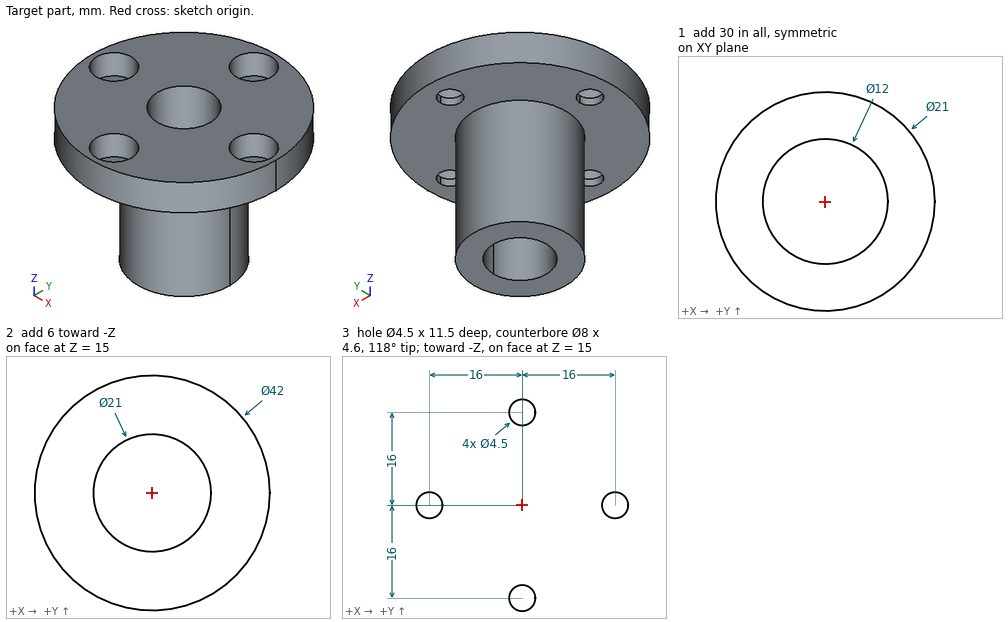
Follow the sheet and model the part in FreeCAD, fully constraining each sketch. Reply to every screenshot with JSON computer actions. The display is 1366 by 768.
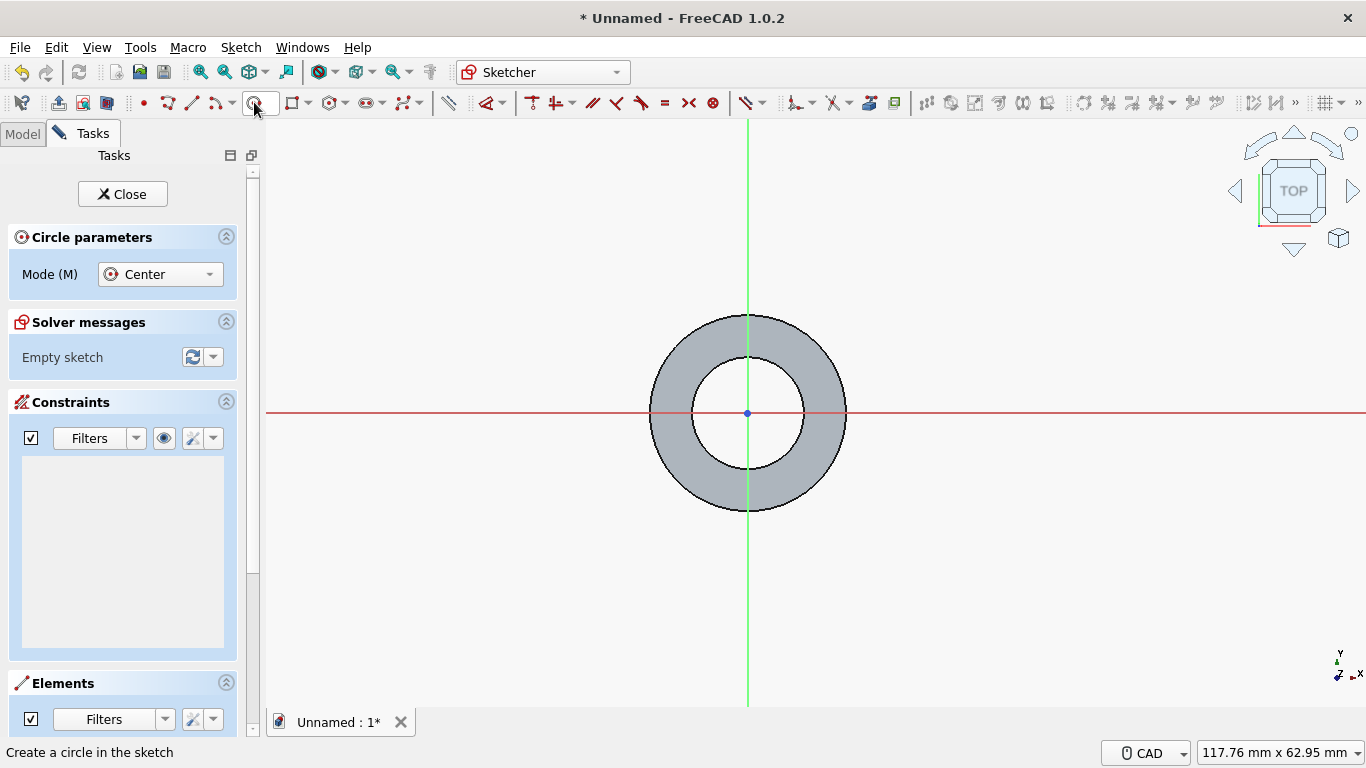
{"action": "left_click", "coordinate": [748, 413]}
{"action": "mouse_move", "coordinate": [887, 274]}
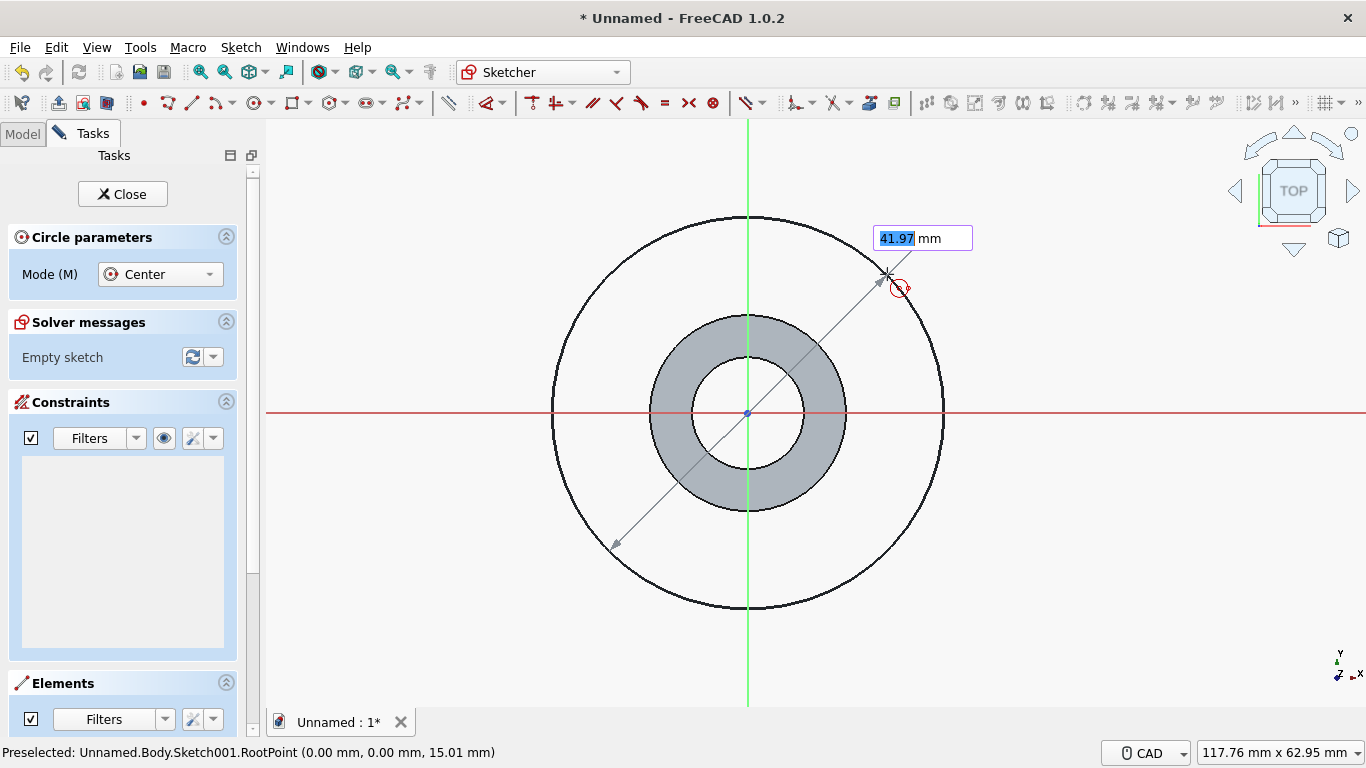
{"action": "type", "text": "42"}
{"action": "key", "text": "Return"}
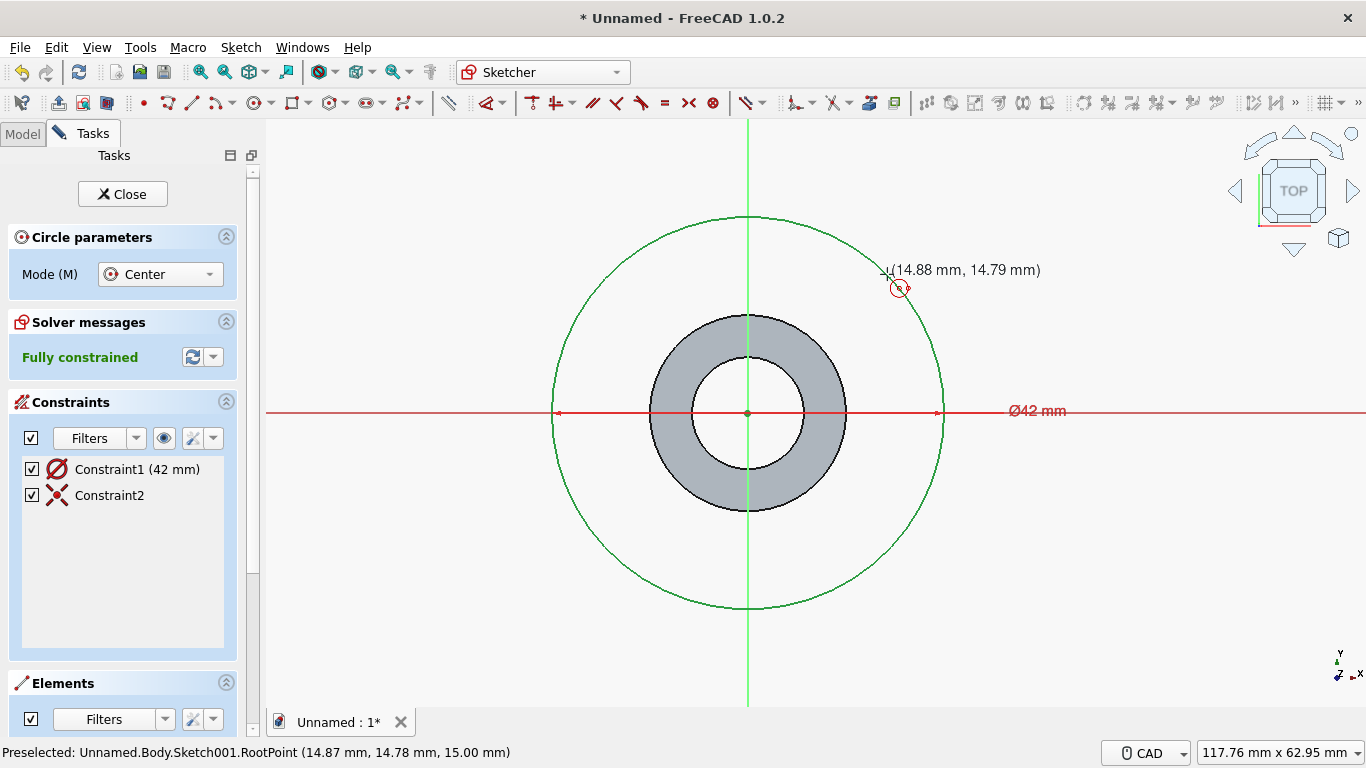
{"action": "left_click", "coordinate": [748, 413]}
{"action": "mouse_move", "coordinate": [817, 344]}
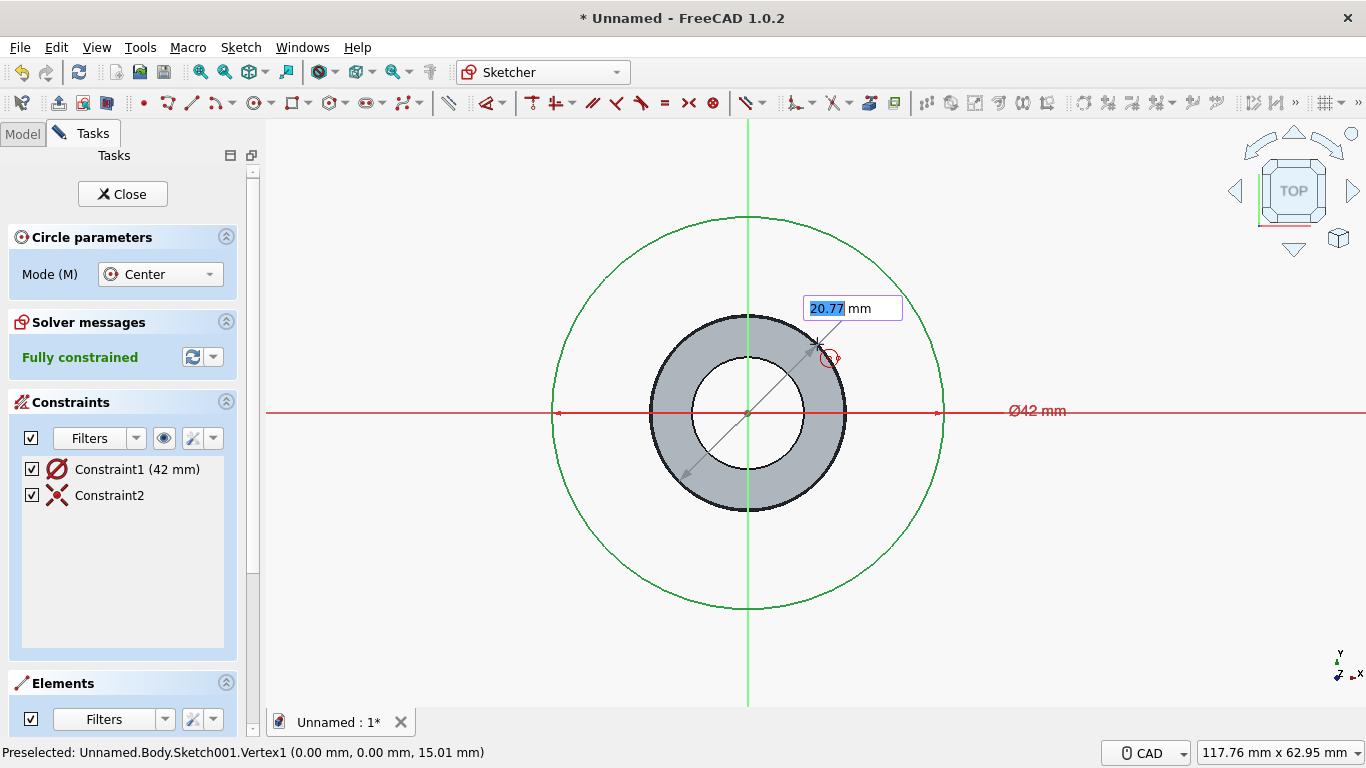
{"action": "type", "text": "21"}
{"action": "key", "text": "Return"}
{"action": "key", "text": "Escape"}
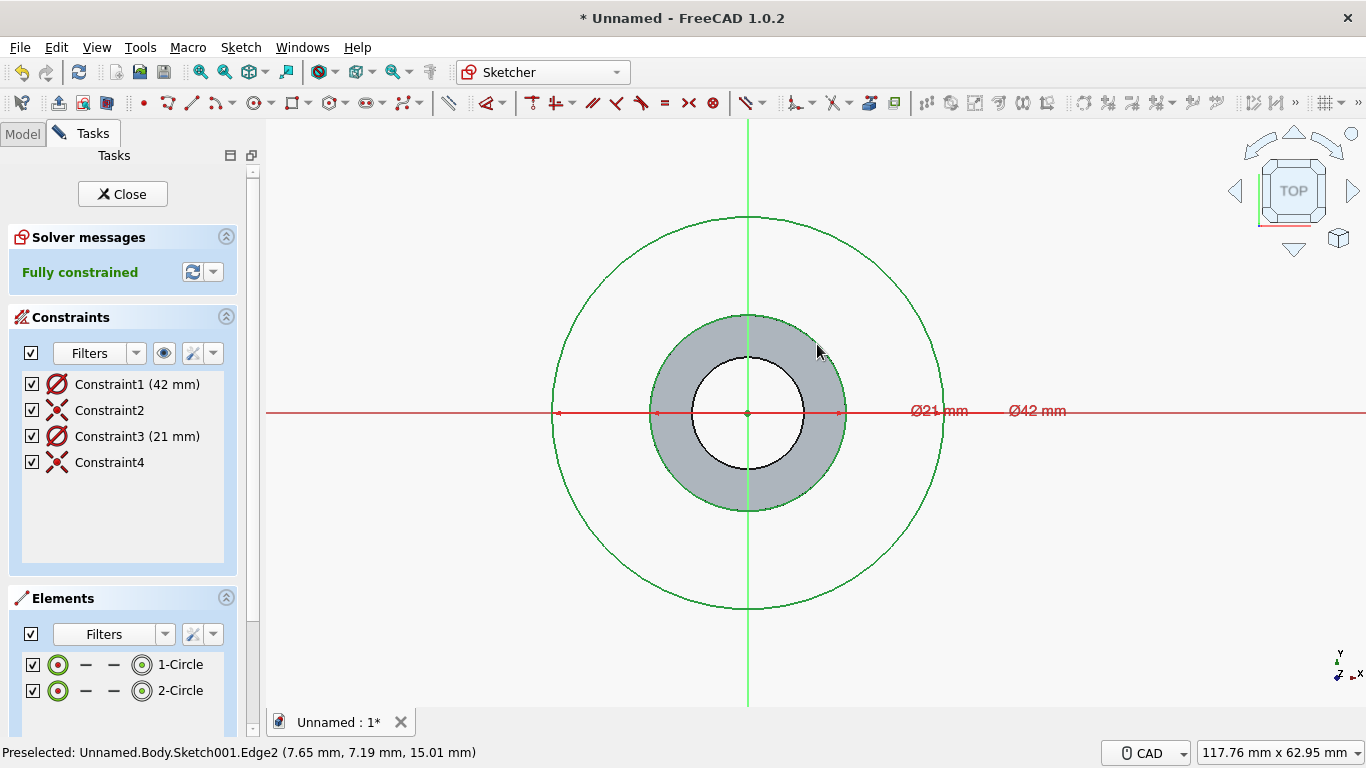
{"action": "left_click", "coordinate": [123, 194]}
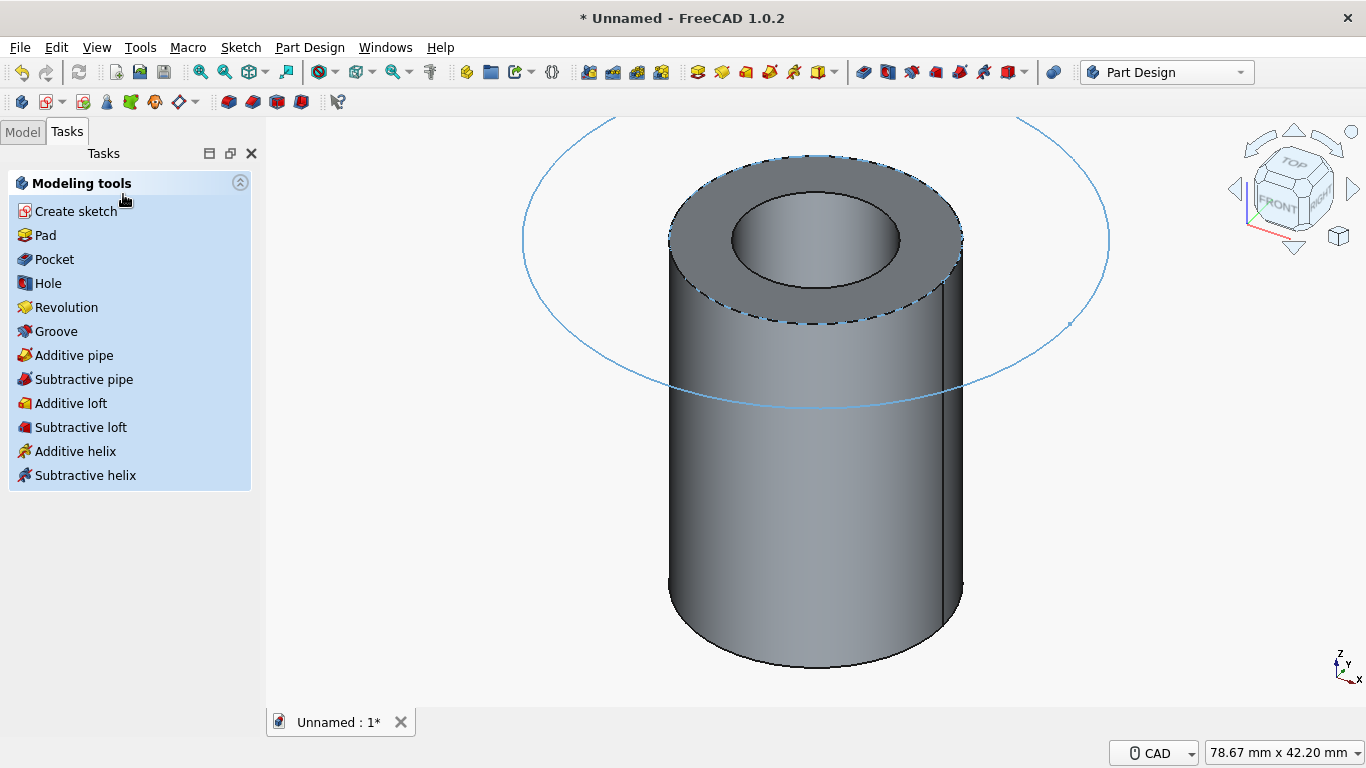
{"action": "left_click", "coordinate": [698, 72]}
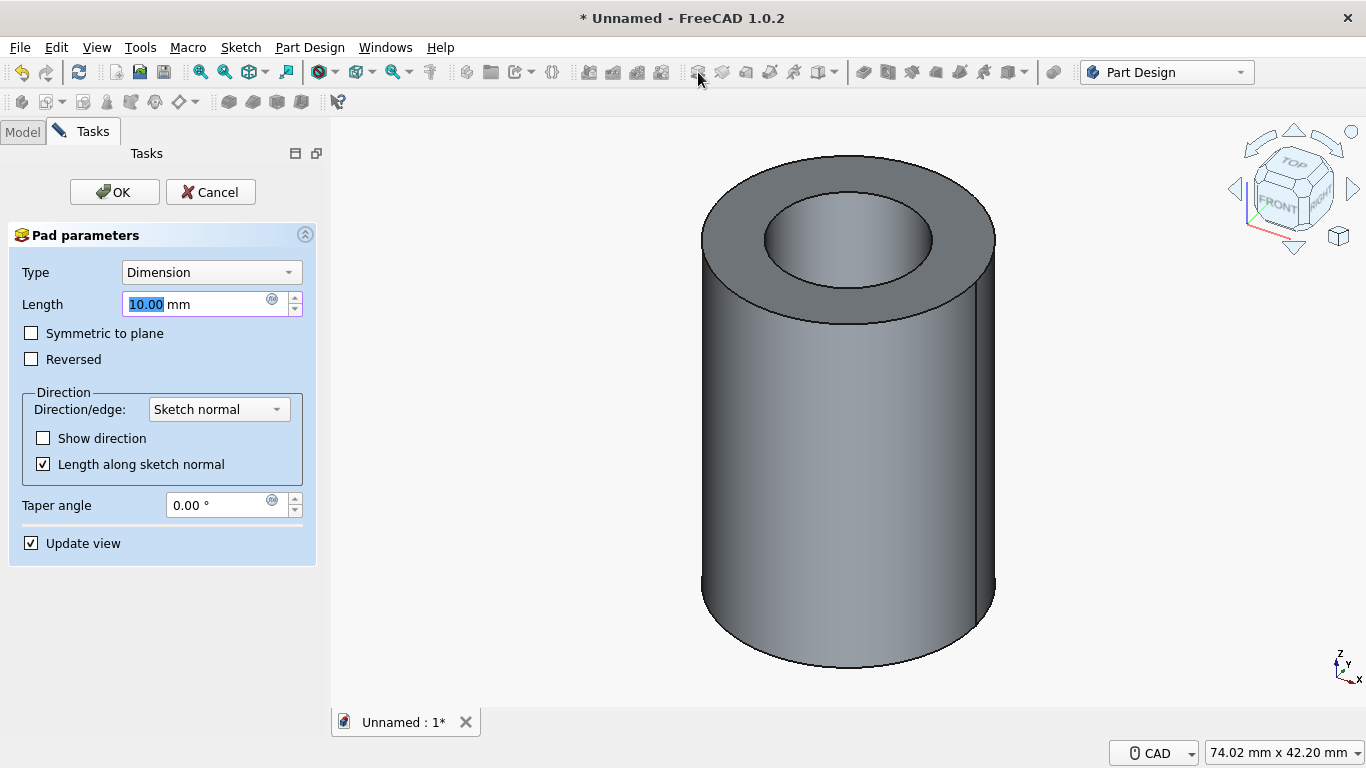
{"action": "type", "text": "6"}
{"action": "key", "text": "Tab"}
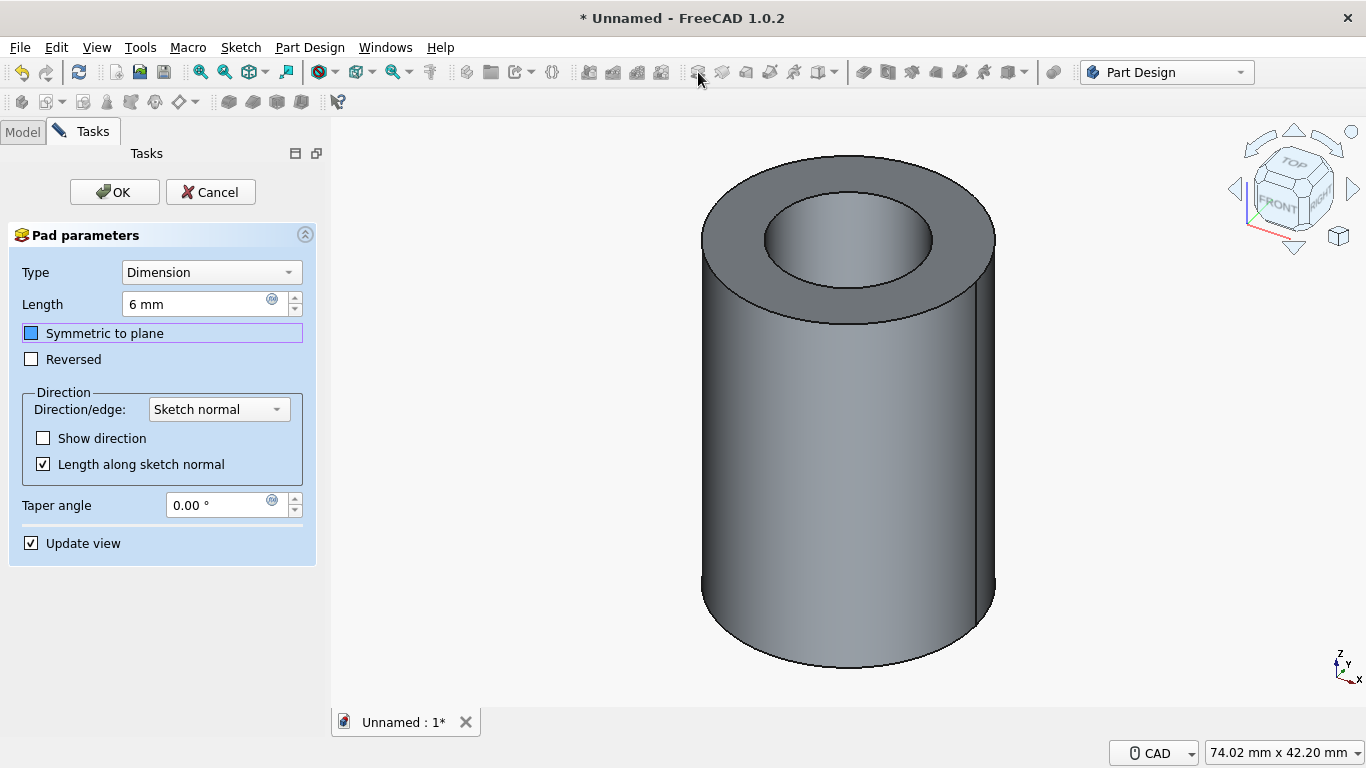
{"action": "left_click", "coordinate": [30, 359]}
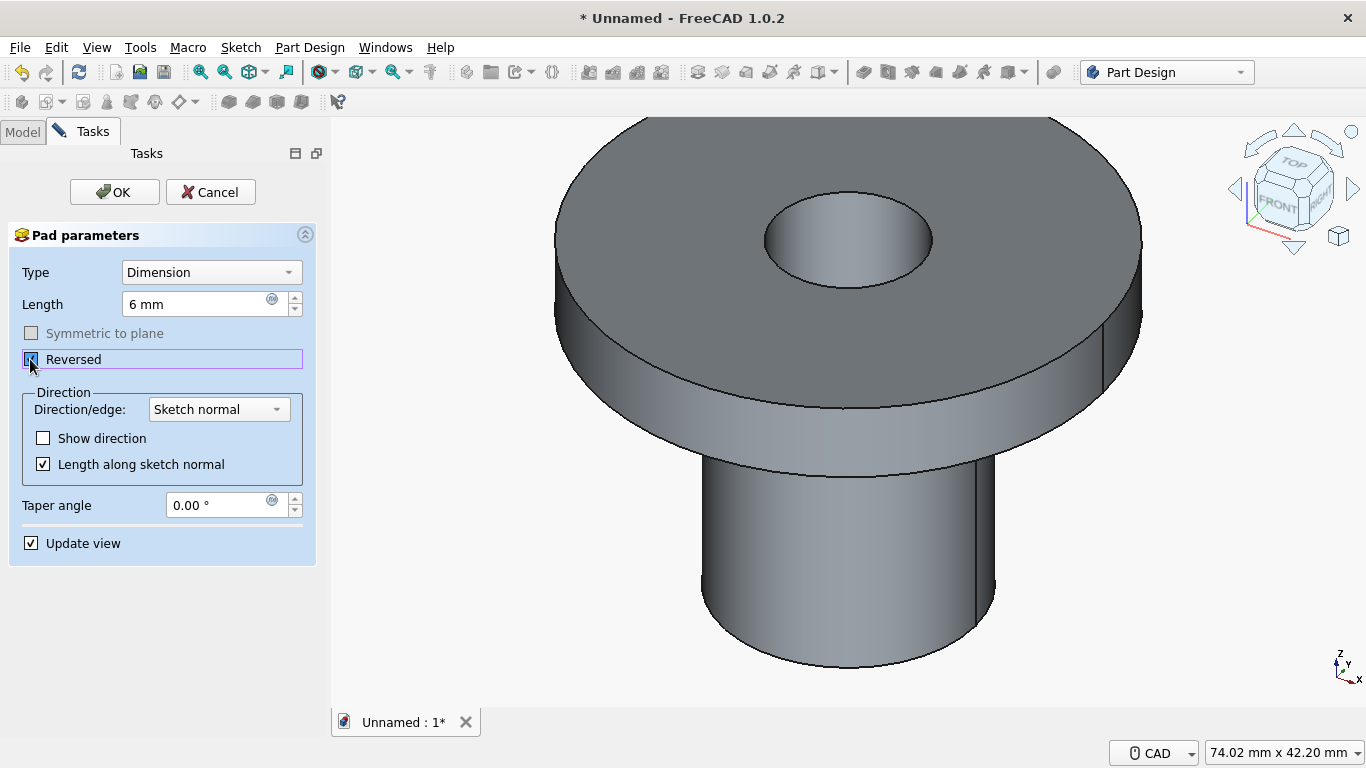
{"action": "left_click", "coordinate": [115, 192]}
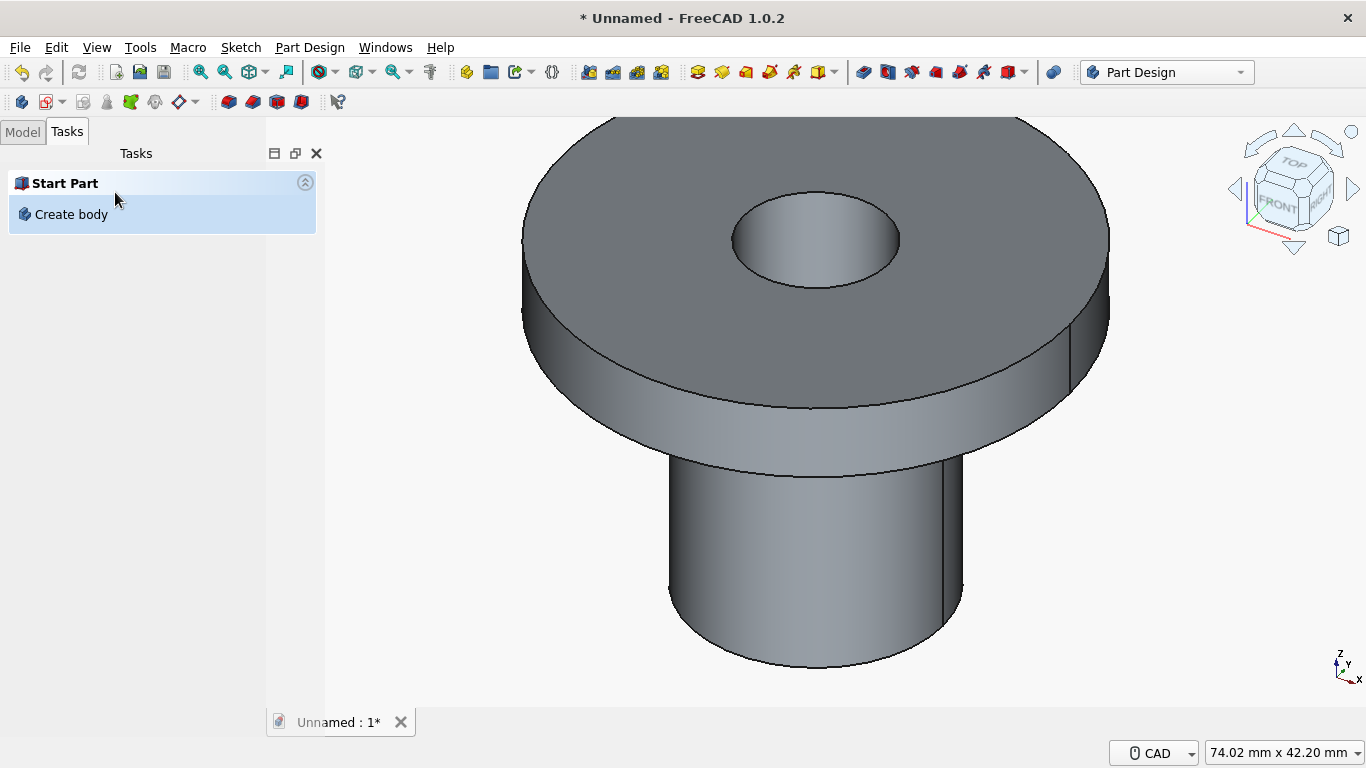
{"action": "left_click", "coordinate": [202, 72]}